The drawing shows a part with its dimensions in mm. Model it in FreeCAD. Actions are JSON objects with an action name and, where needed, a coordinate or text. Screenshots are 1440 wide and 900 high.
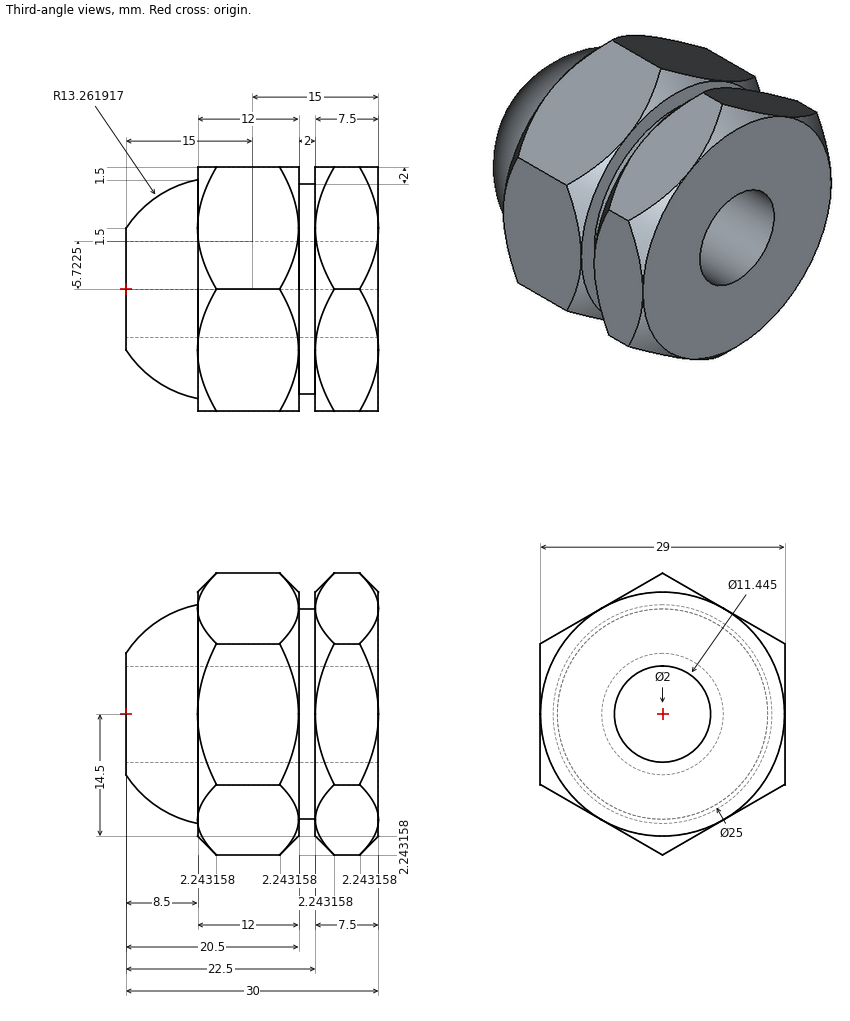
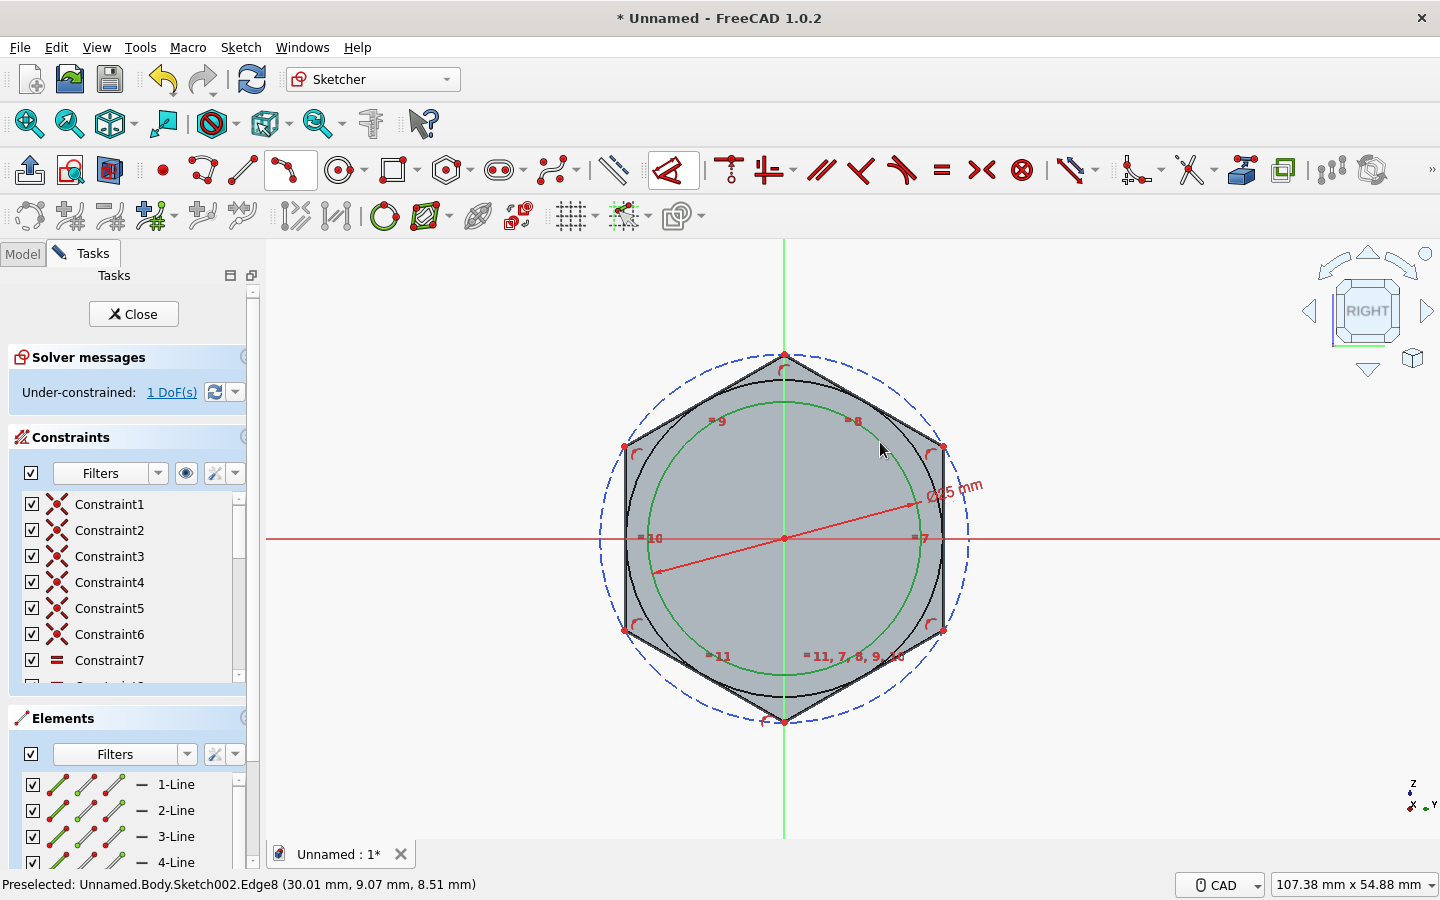
{"action": "left_click", "coordinate": [625, 446]}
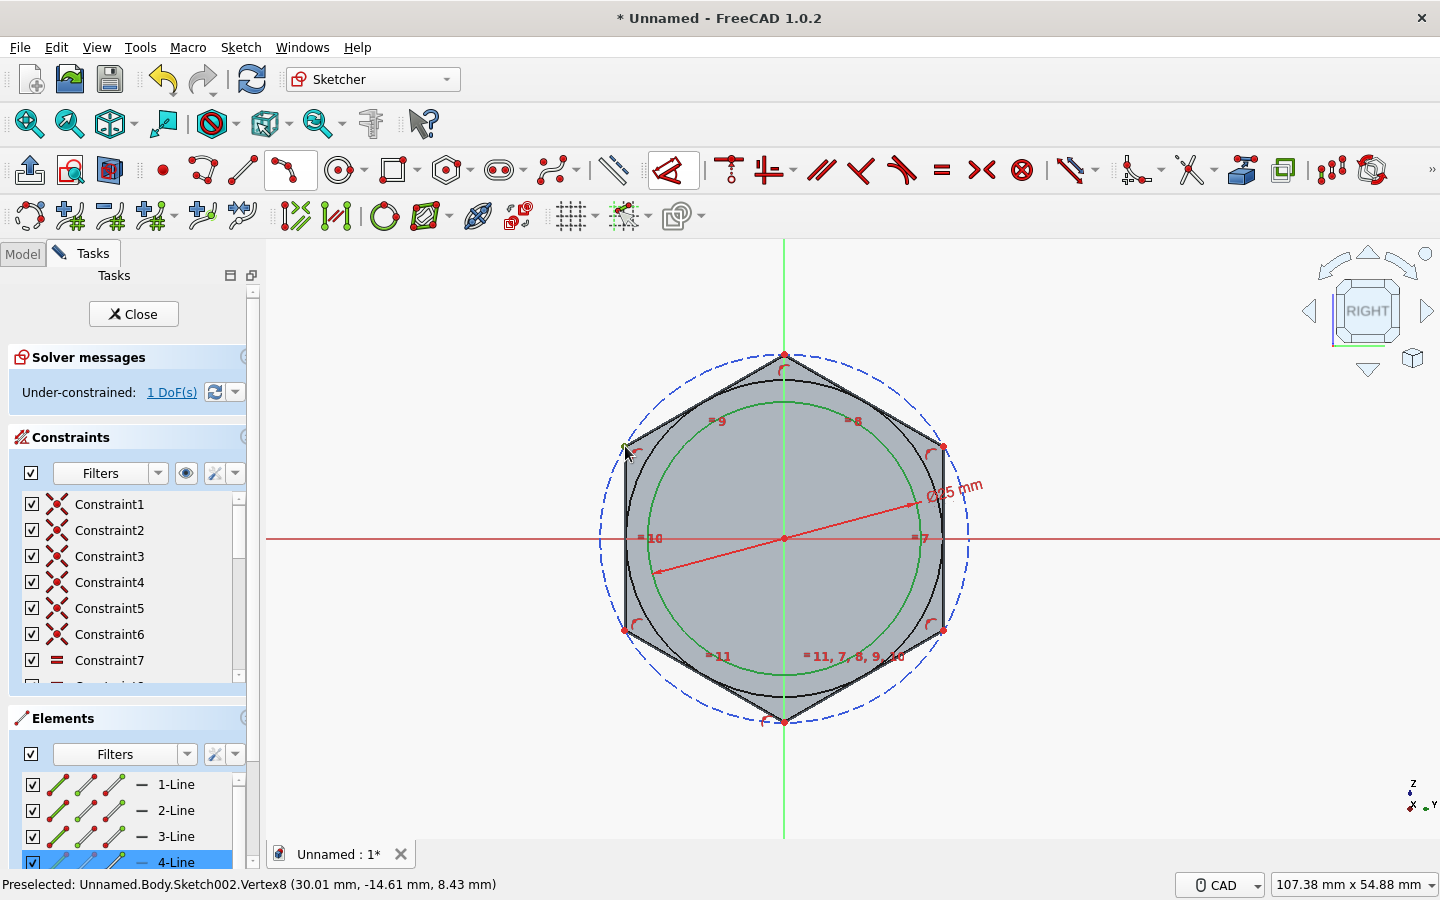
{"action": "left_click", "coordinate": [944, 631]}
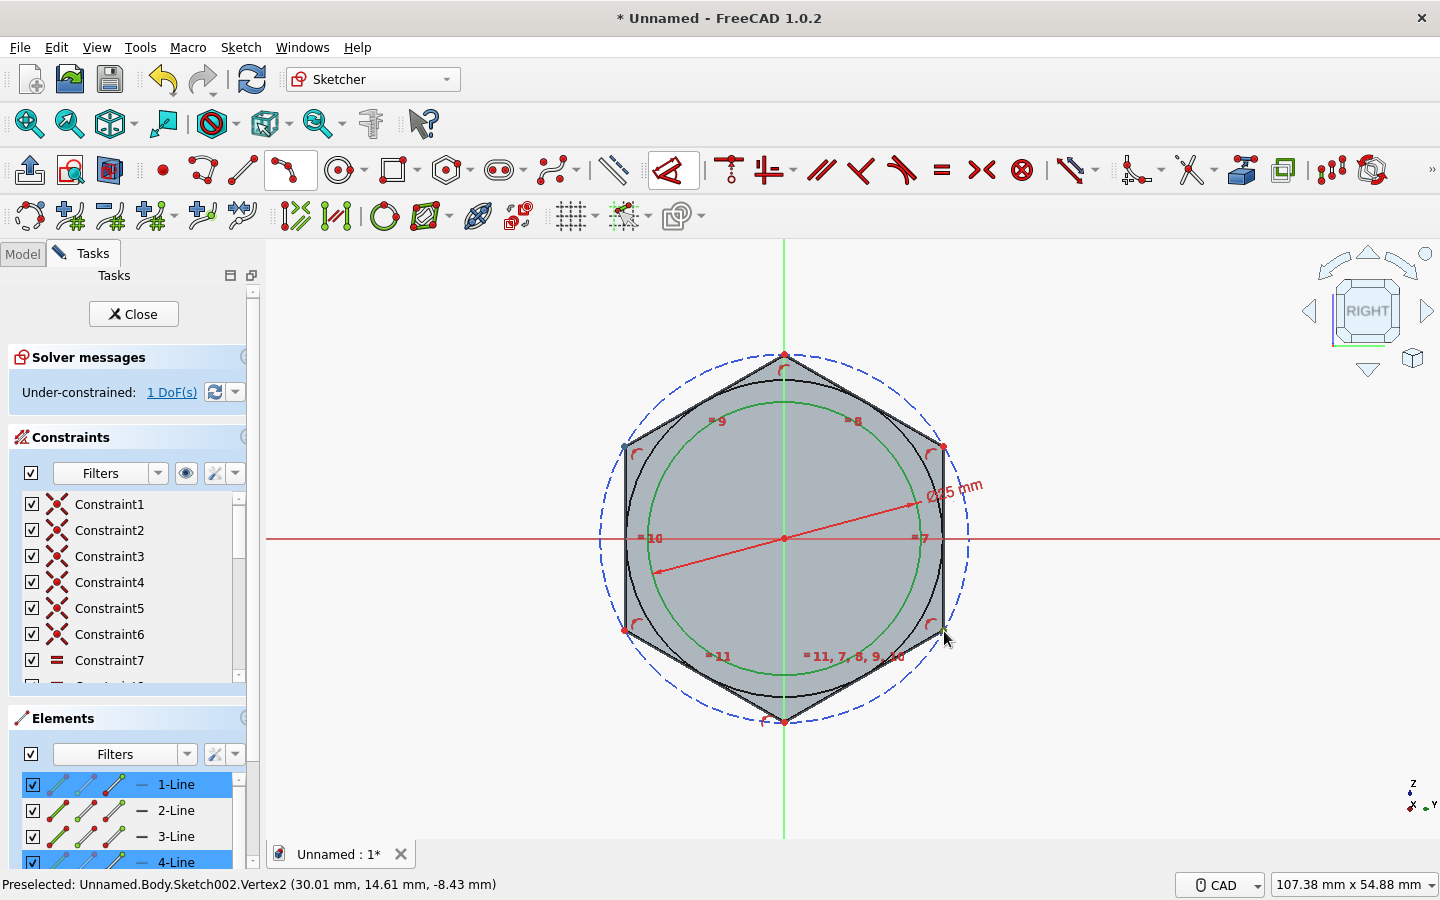
{"action": "key", "text": "l"}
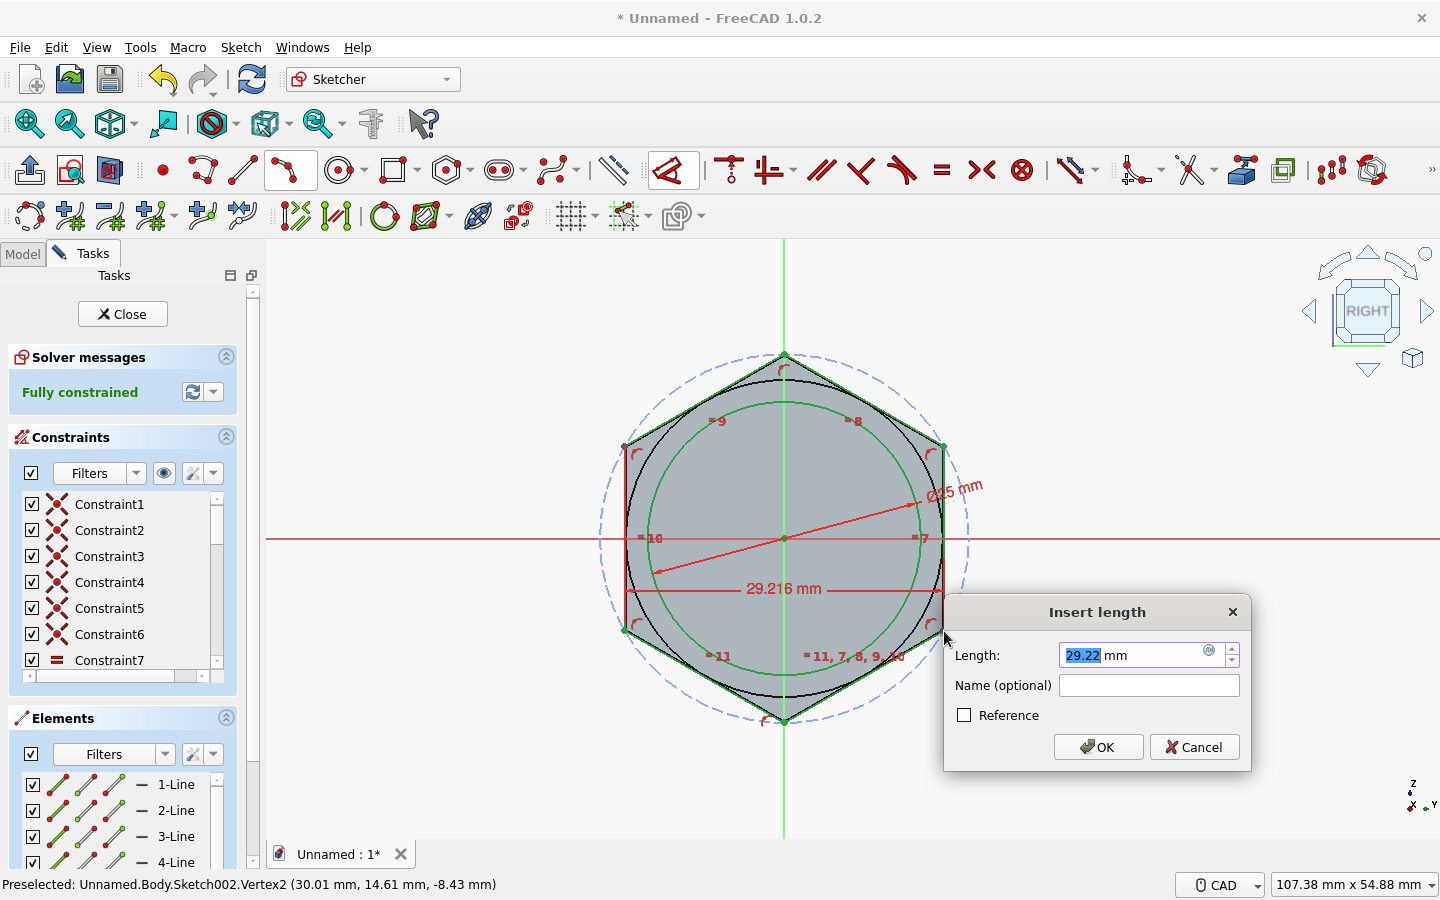
{"action": "type", "text": "29"}
{"action": "key", "text": "Return"}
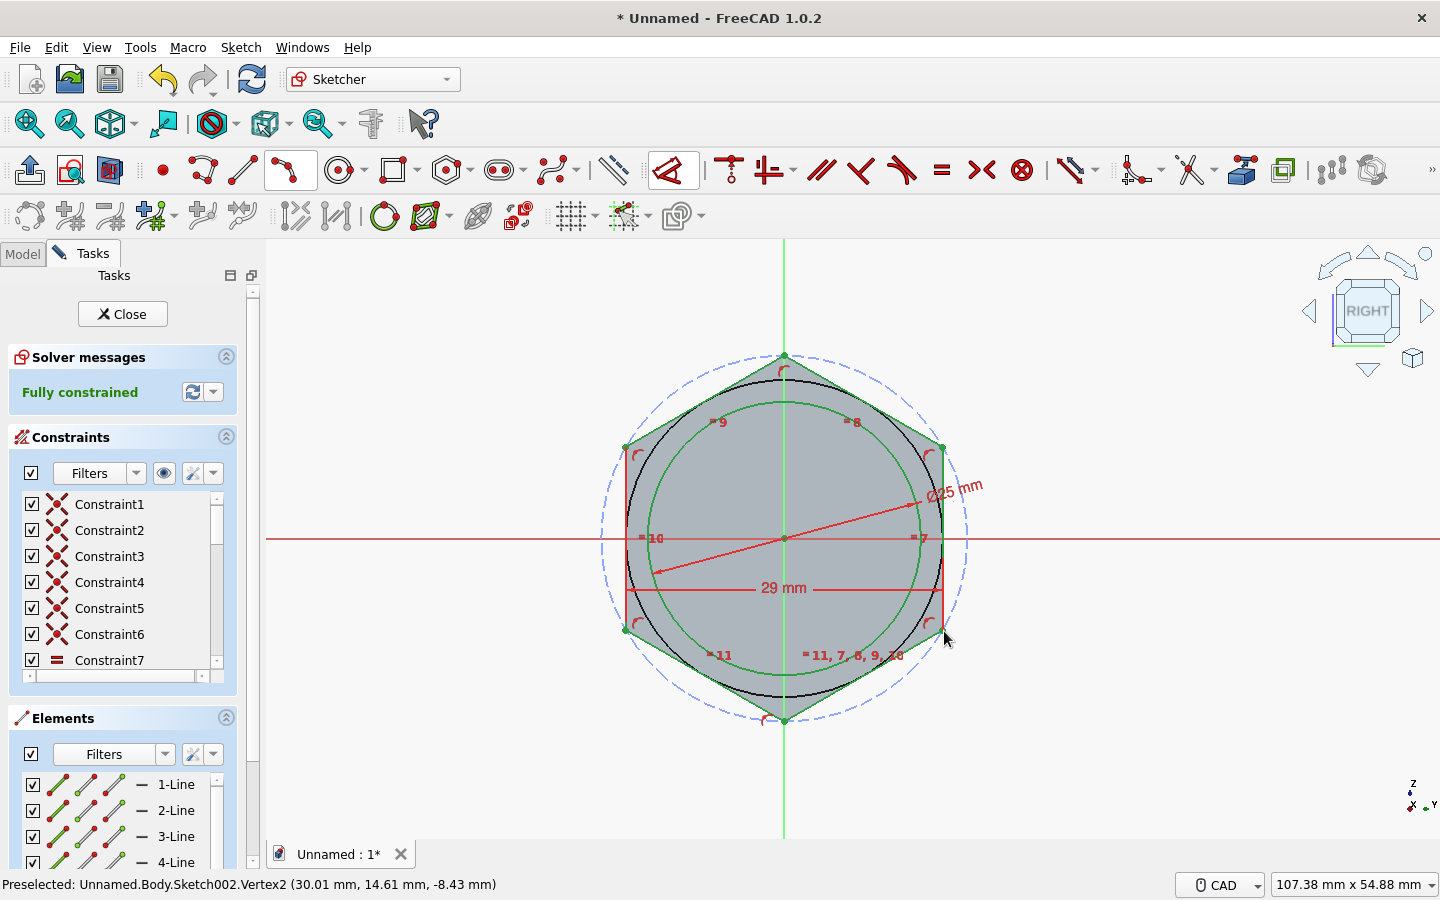
{"action": "left_click", "coordinate": [123, 314]}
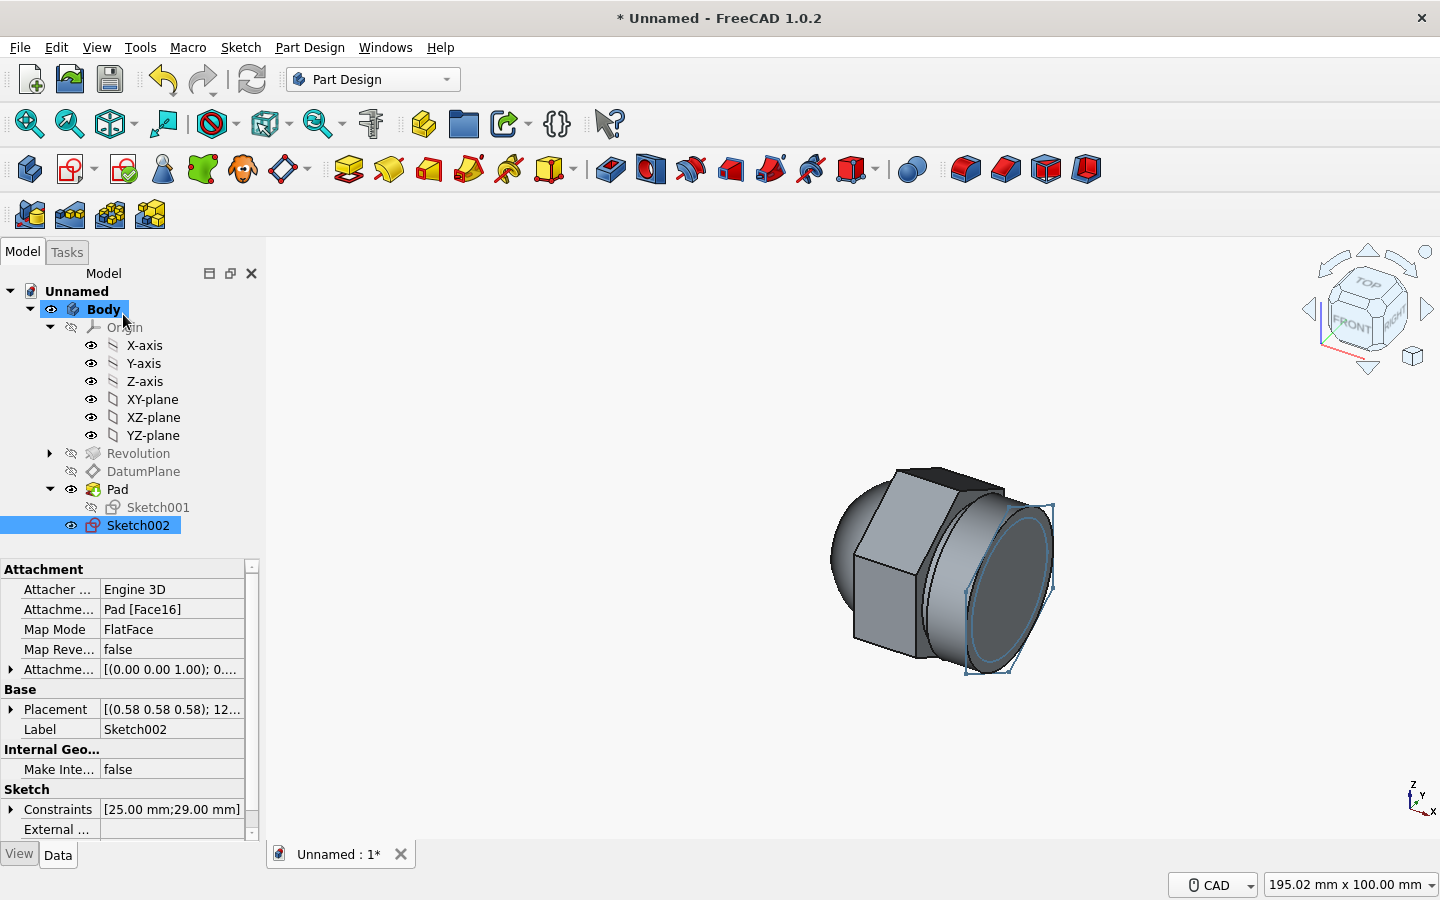
{"action": "left_click", "coordinate": [350, 170]}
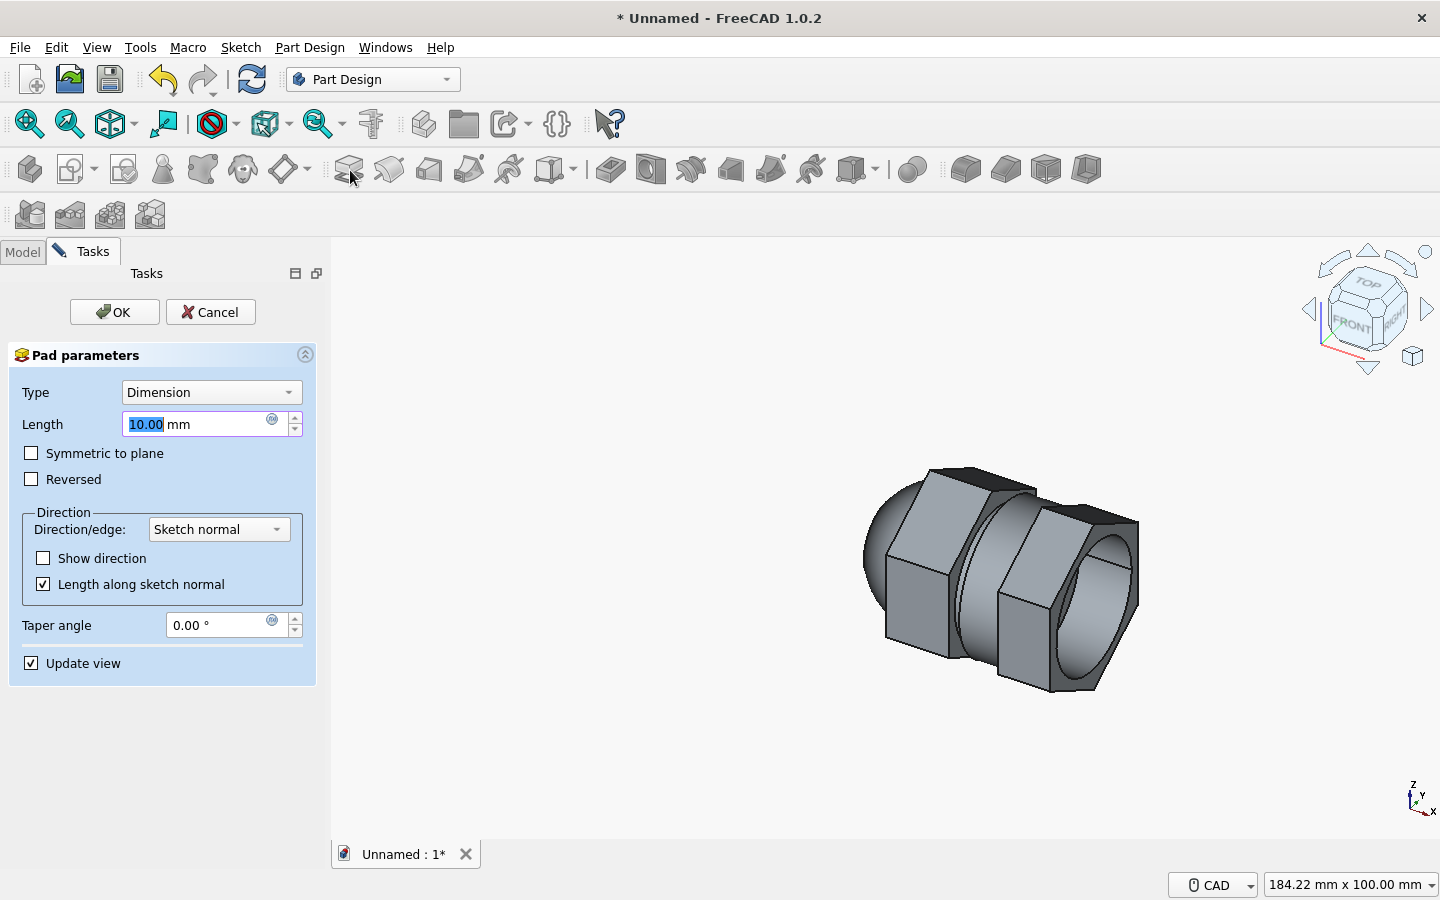
{"action": "type", "text": "7.5"}
{"action": "key", "text": "Tab"}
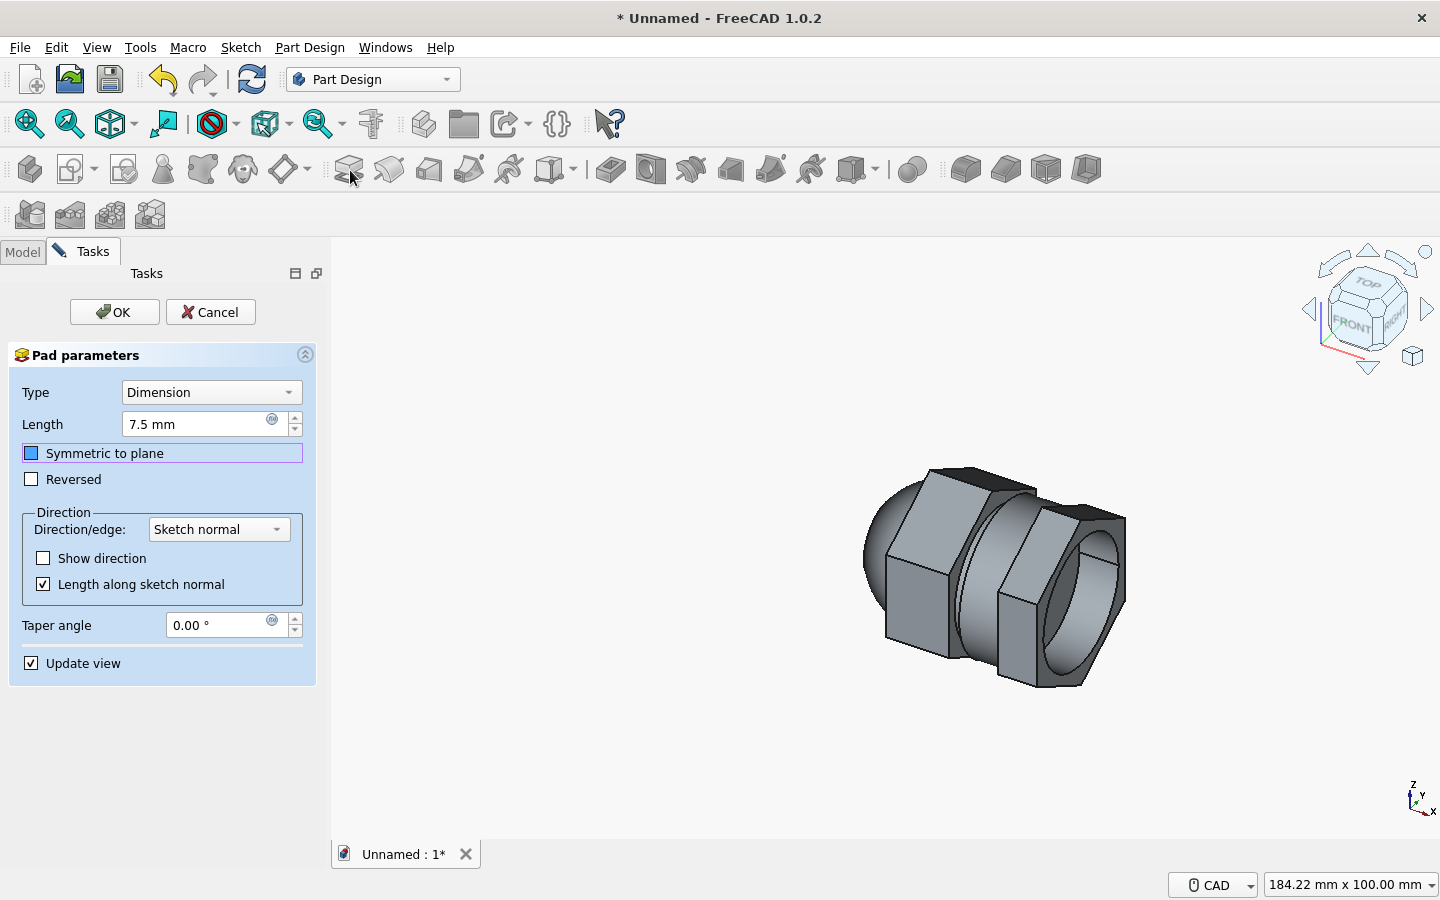
{"action": "left_click", "coordinate": [30, 479]}